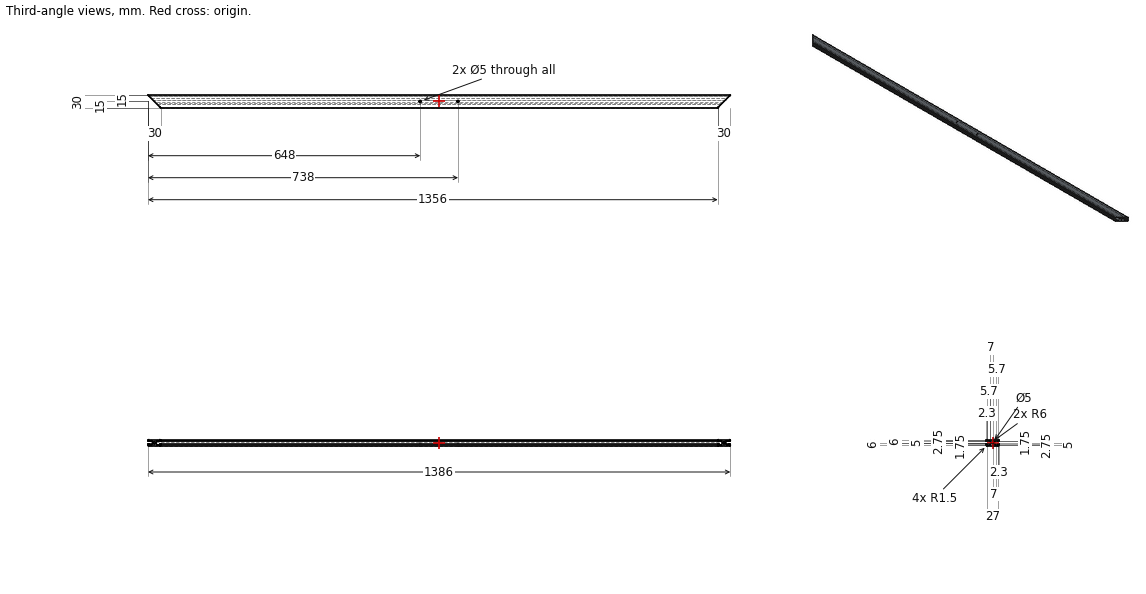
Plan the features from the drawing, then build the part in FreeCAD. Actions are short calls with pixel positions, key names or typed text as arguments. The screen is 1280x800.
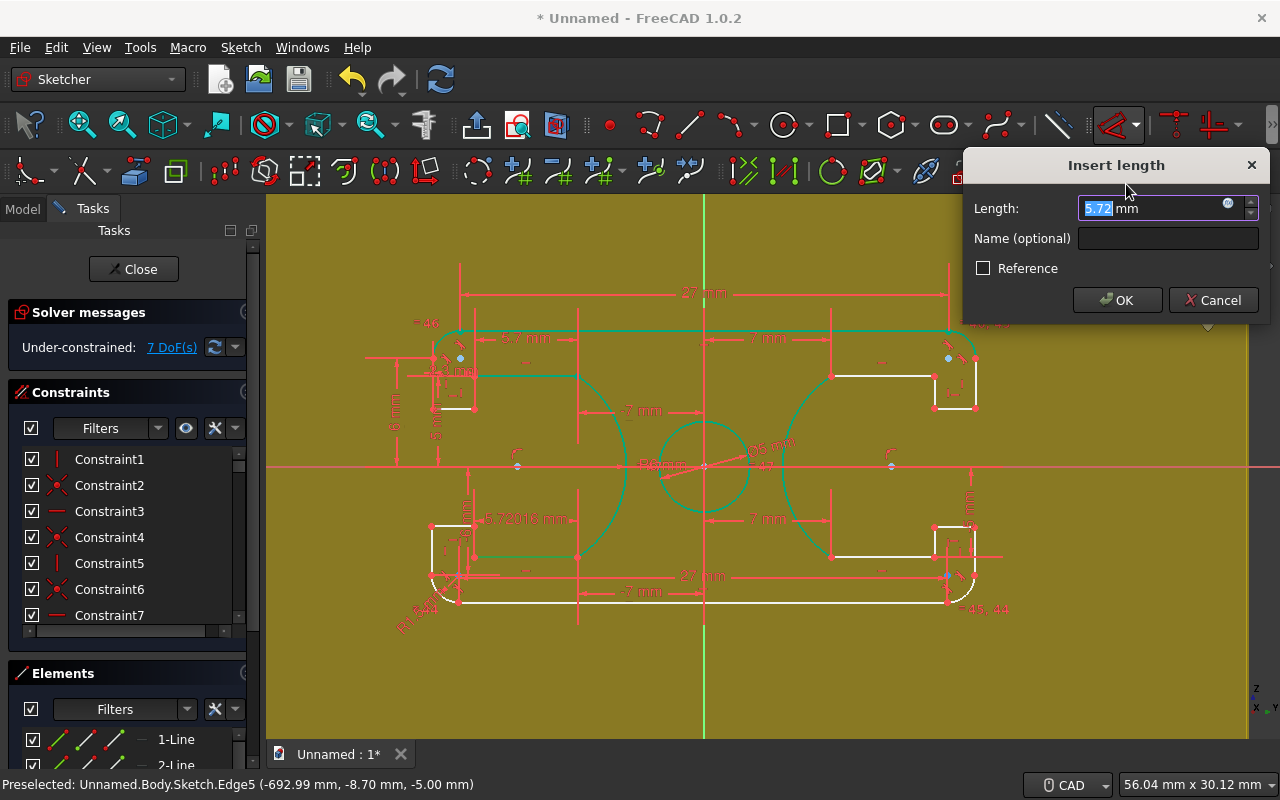
text(5.7)
key(Return)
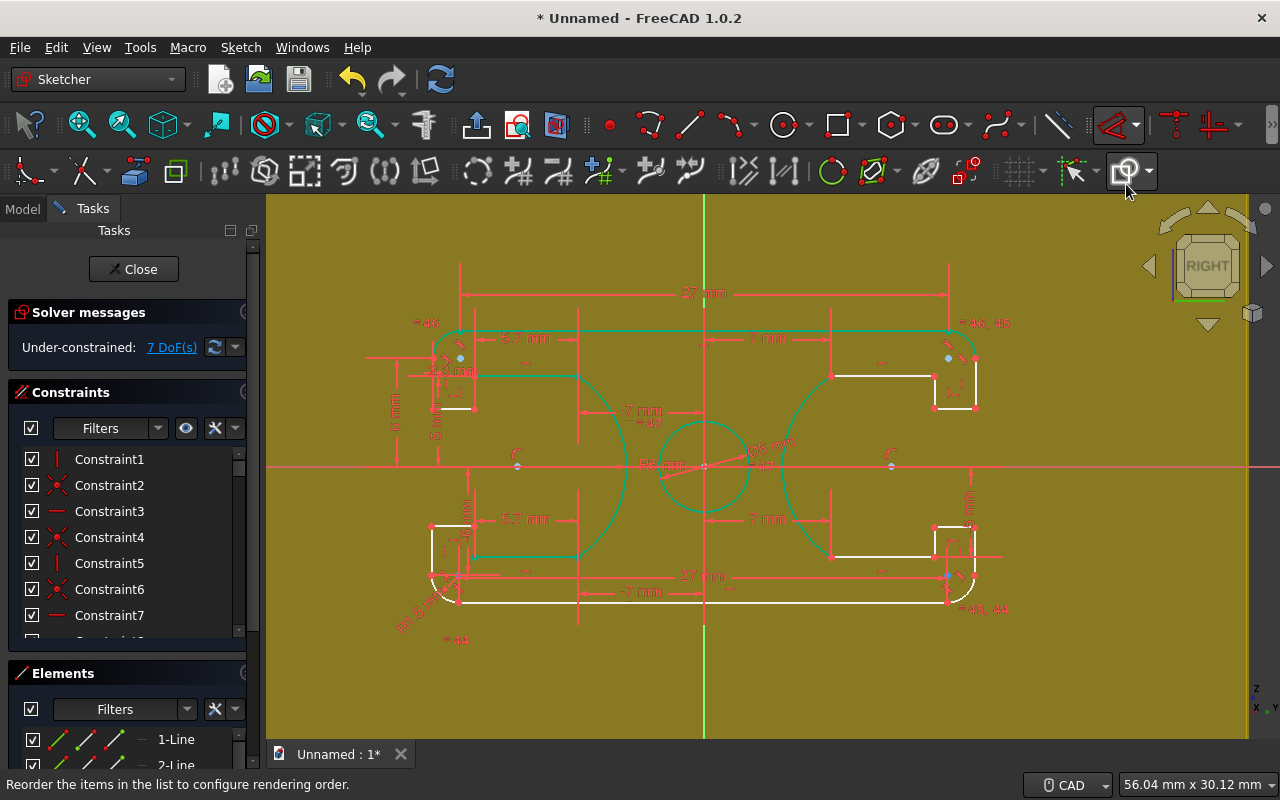
click(445, 526)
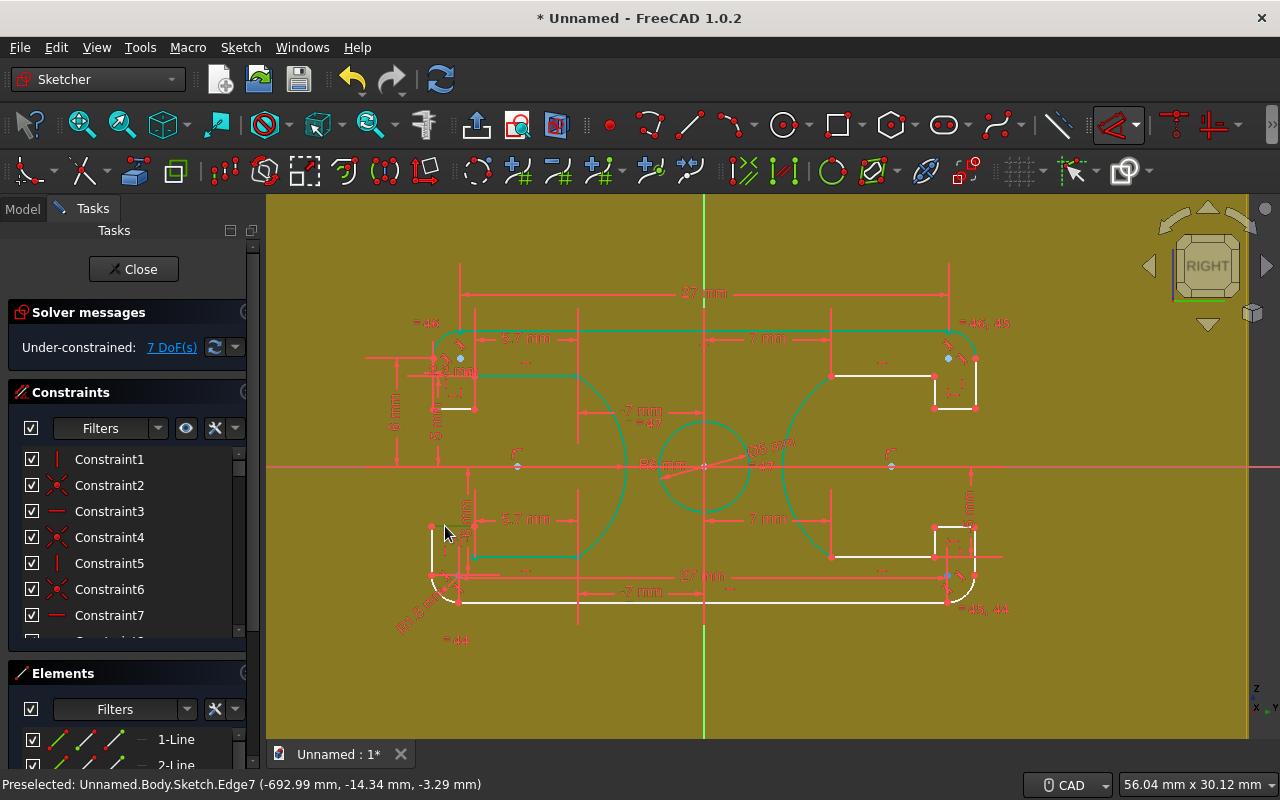
click(1138, 126)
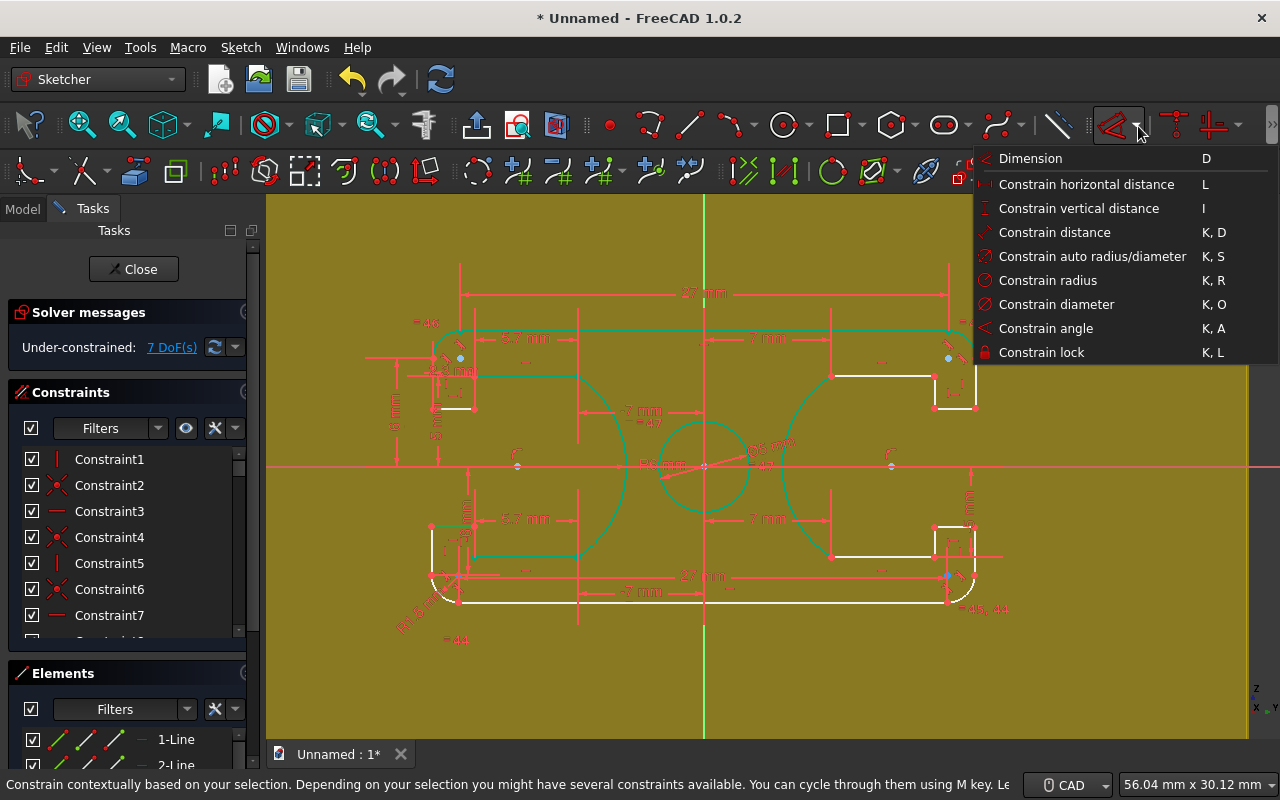
click(1126, 184)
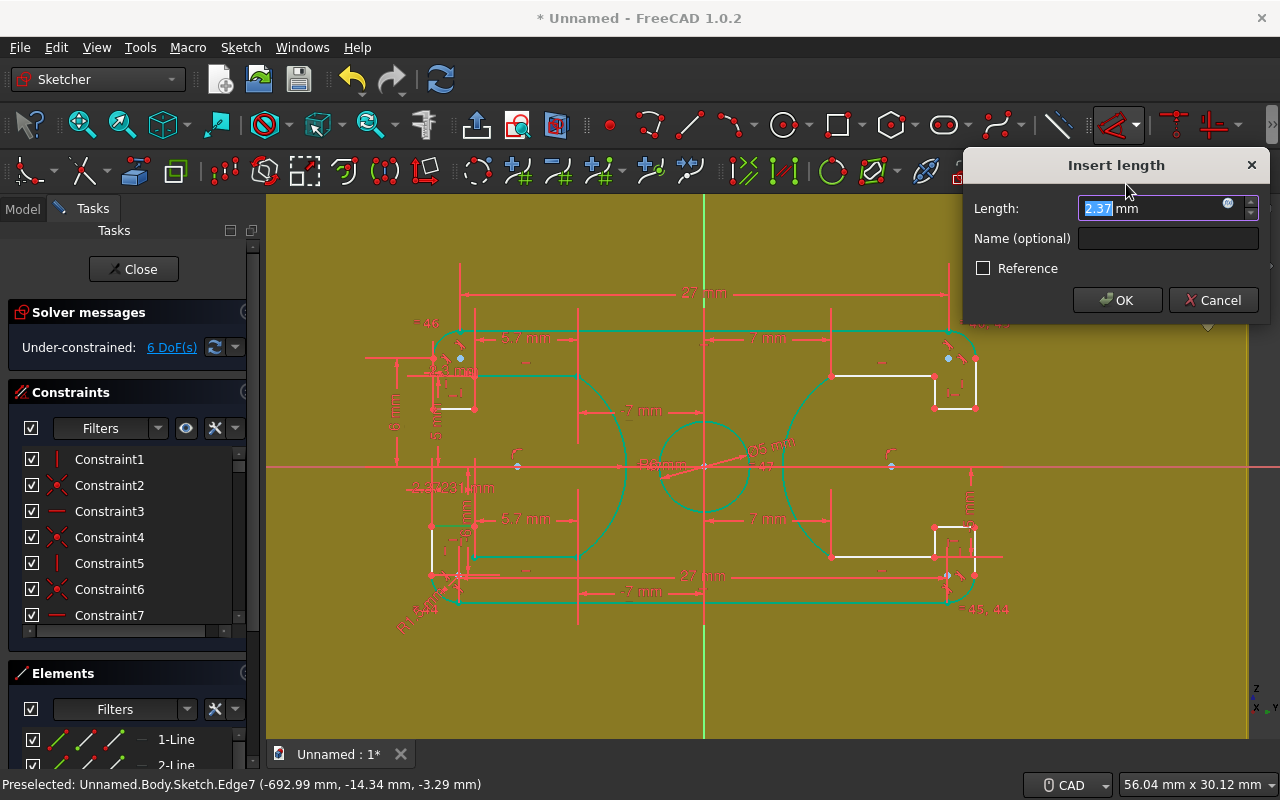
text(2.3)
key(Return)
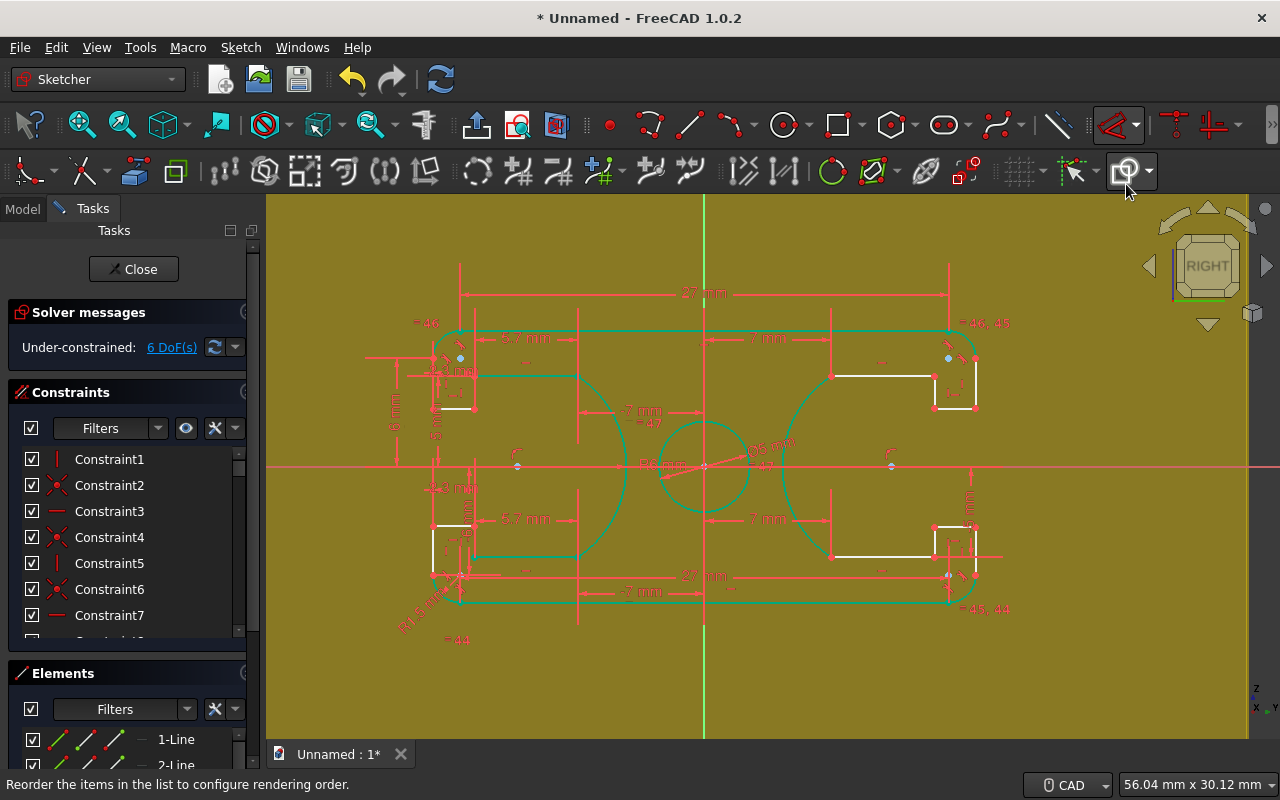
click(947, 527)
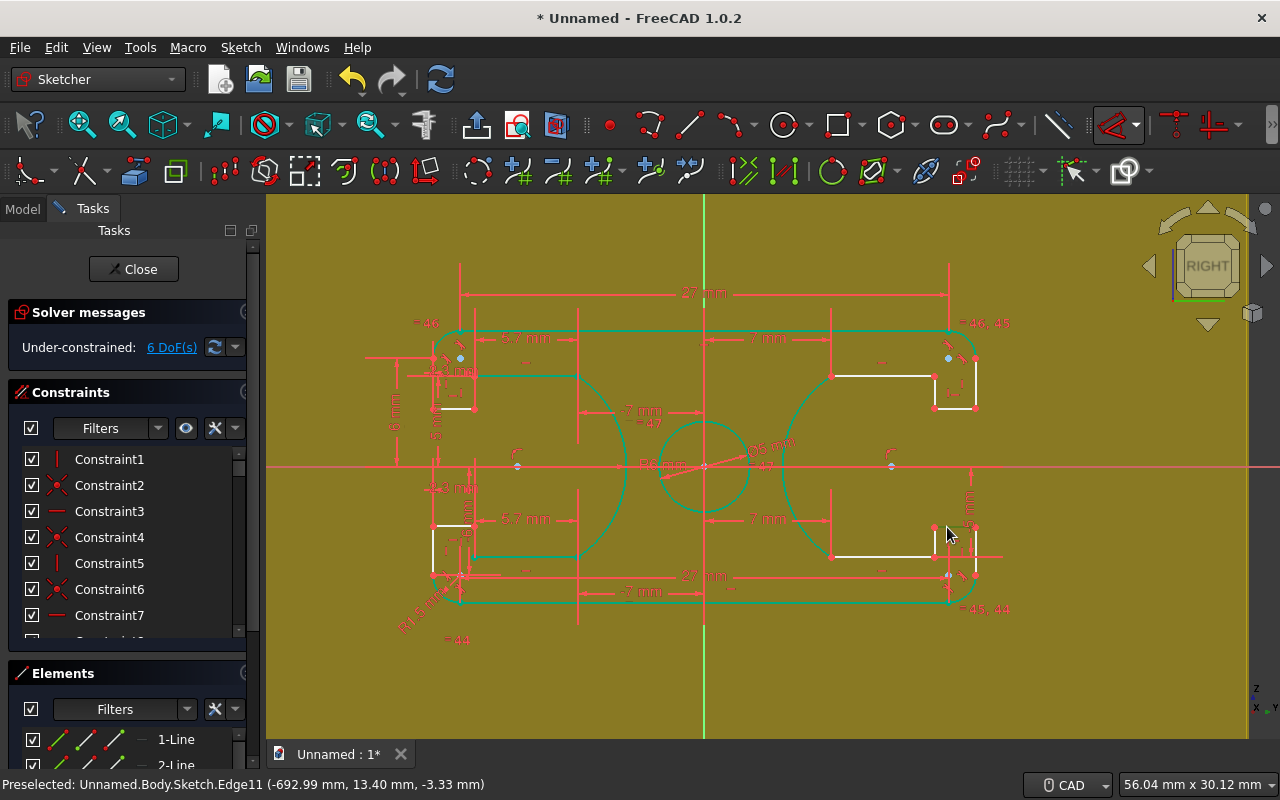
key(l)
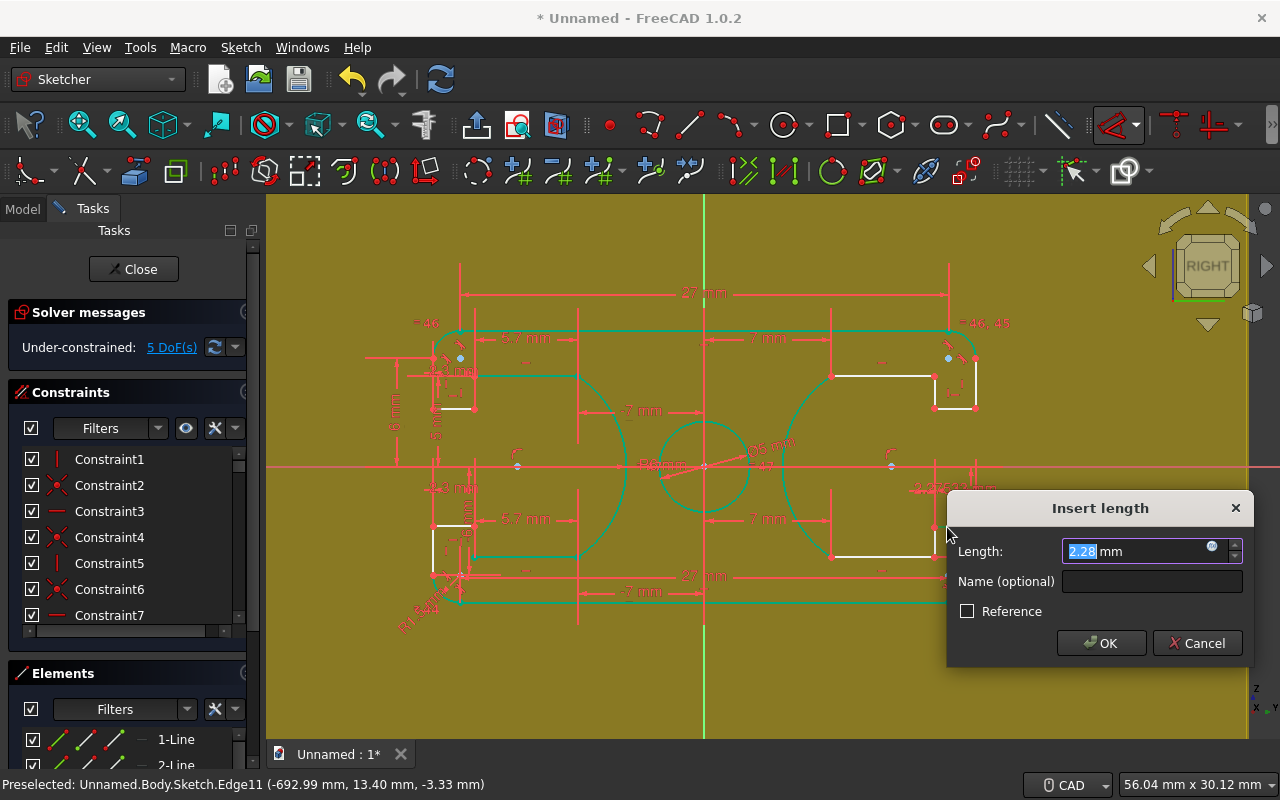
text(2.3)
key(Return)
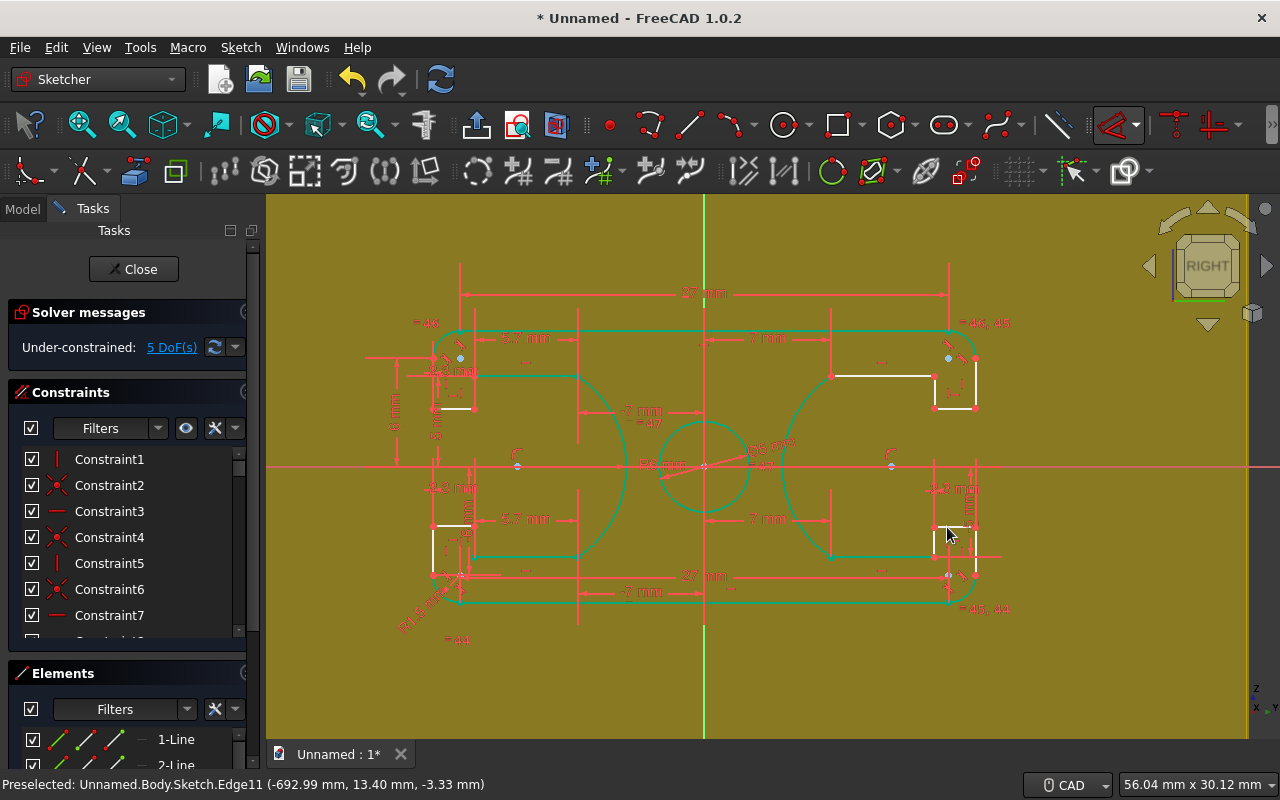
click(862, 376)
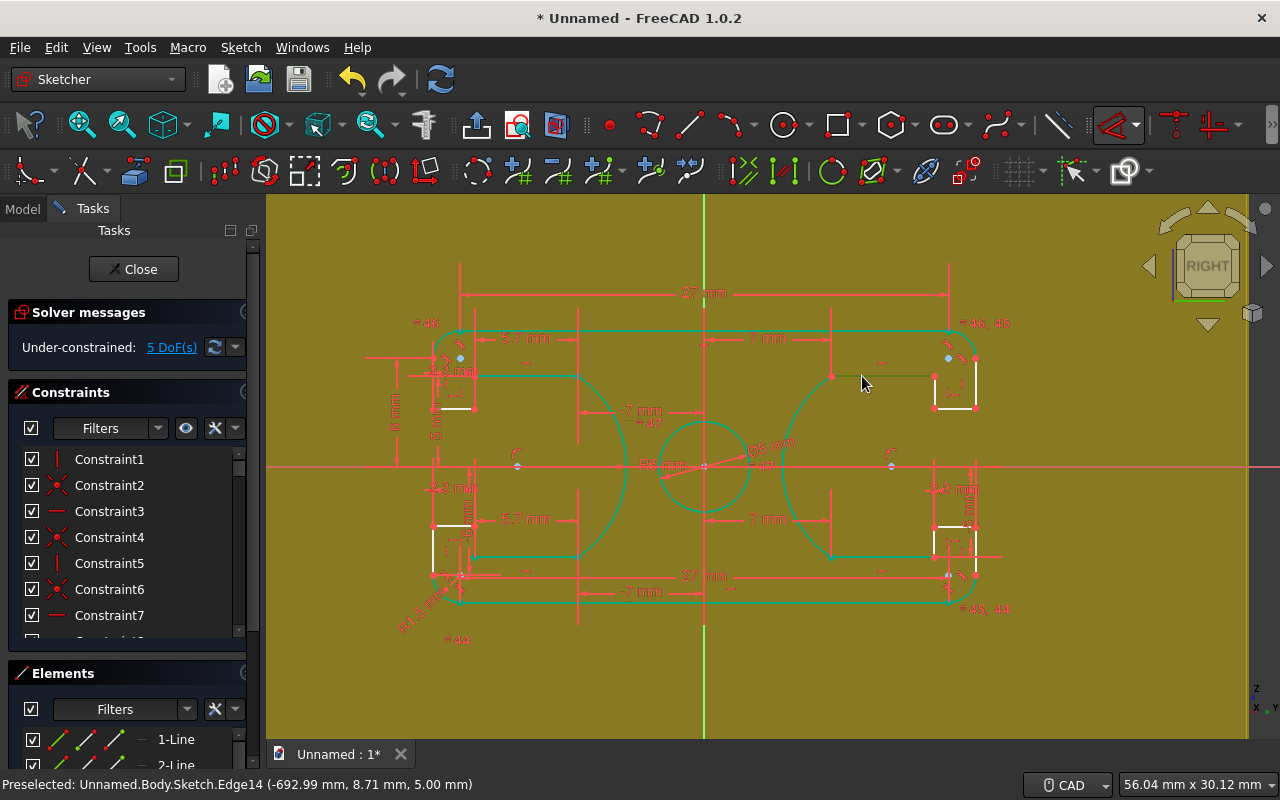
click(1138, 126)